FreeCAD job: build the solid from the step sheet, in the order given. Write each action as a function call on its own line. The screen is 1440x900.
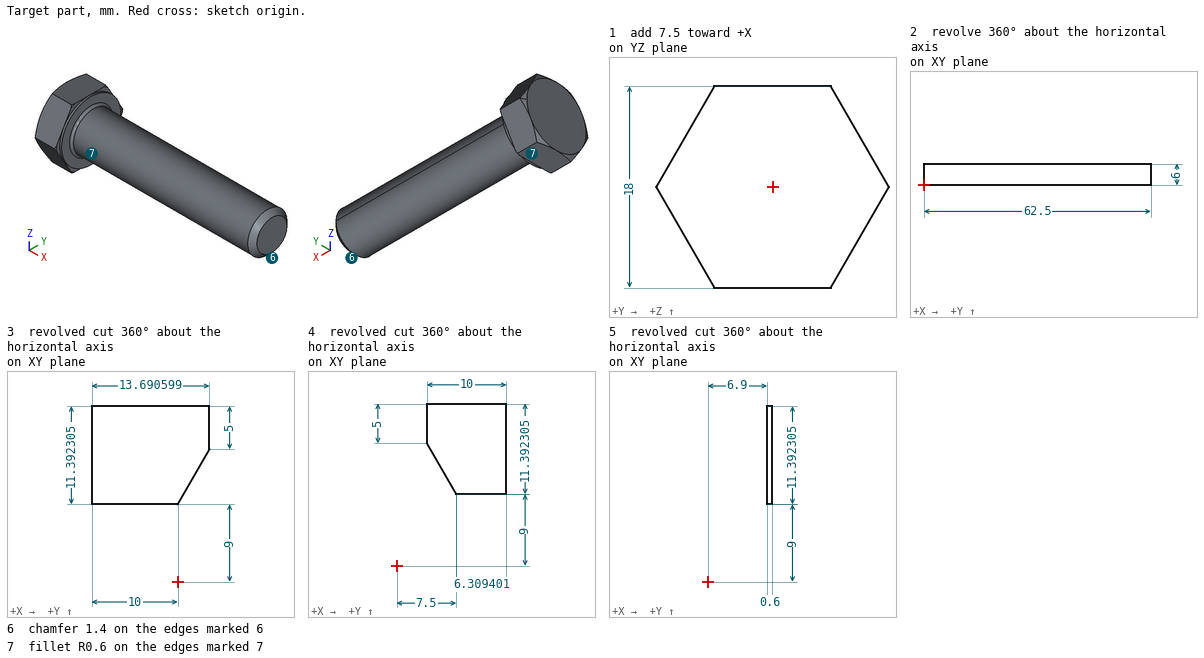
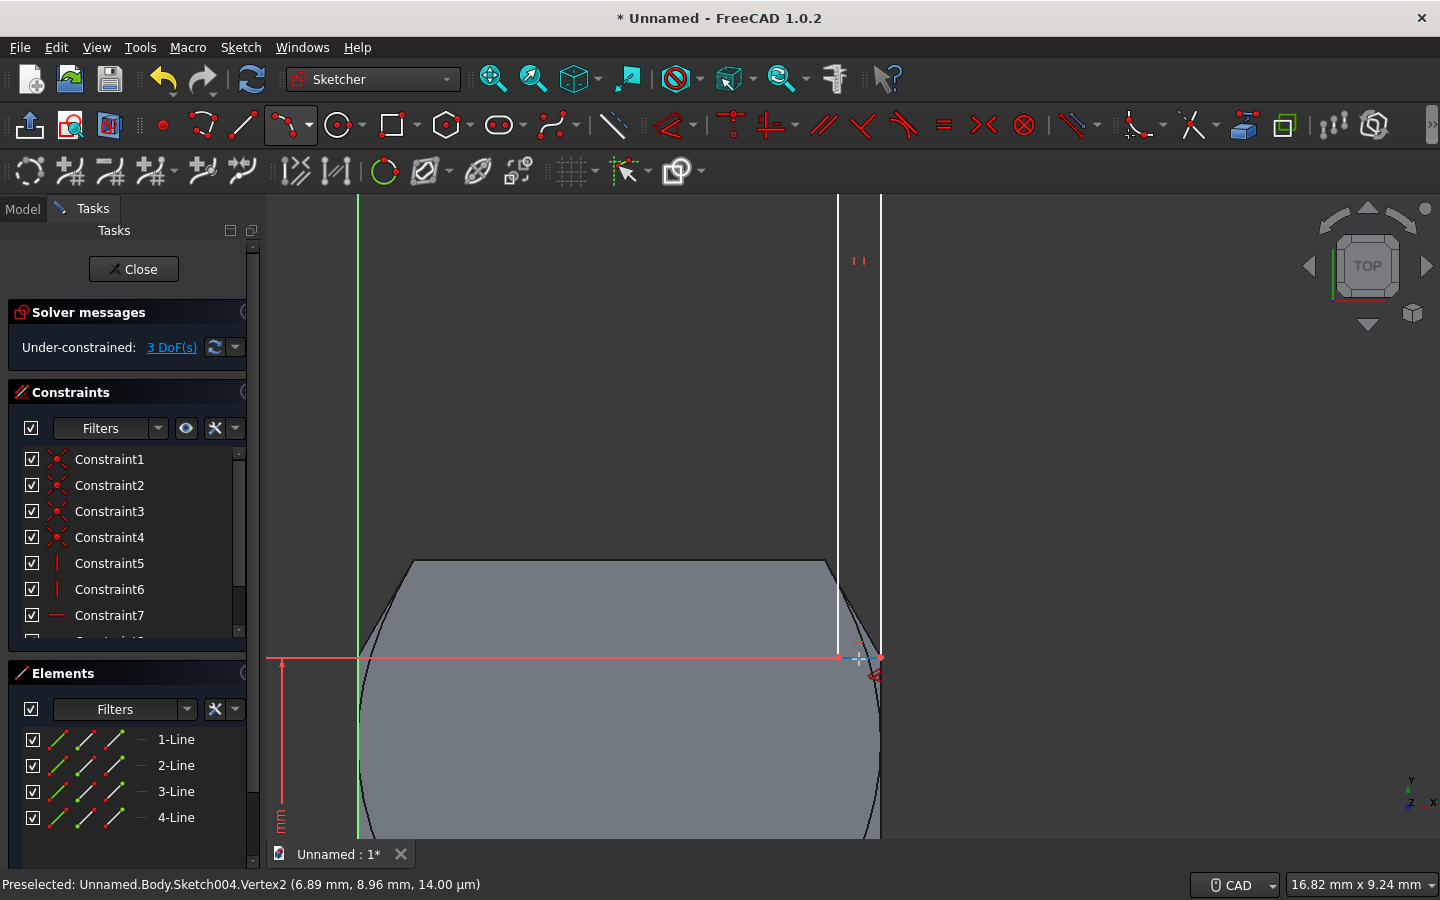
click(859, 658)
click(859, 692)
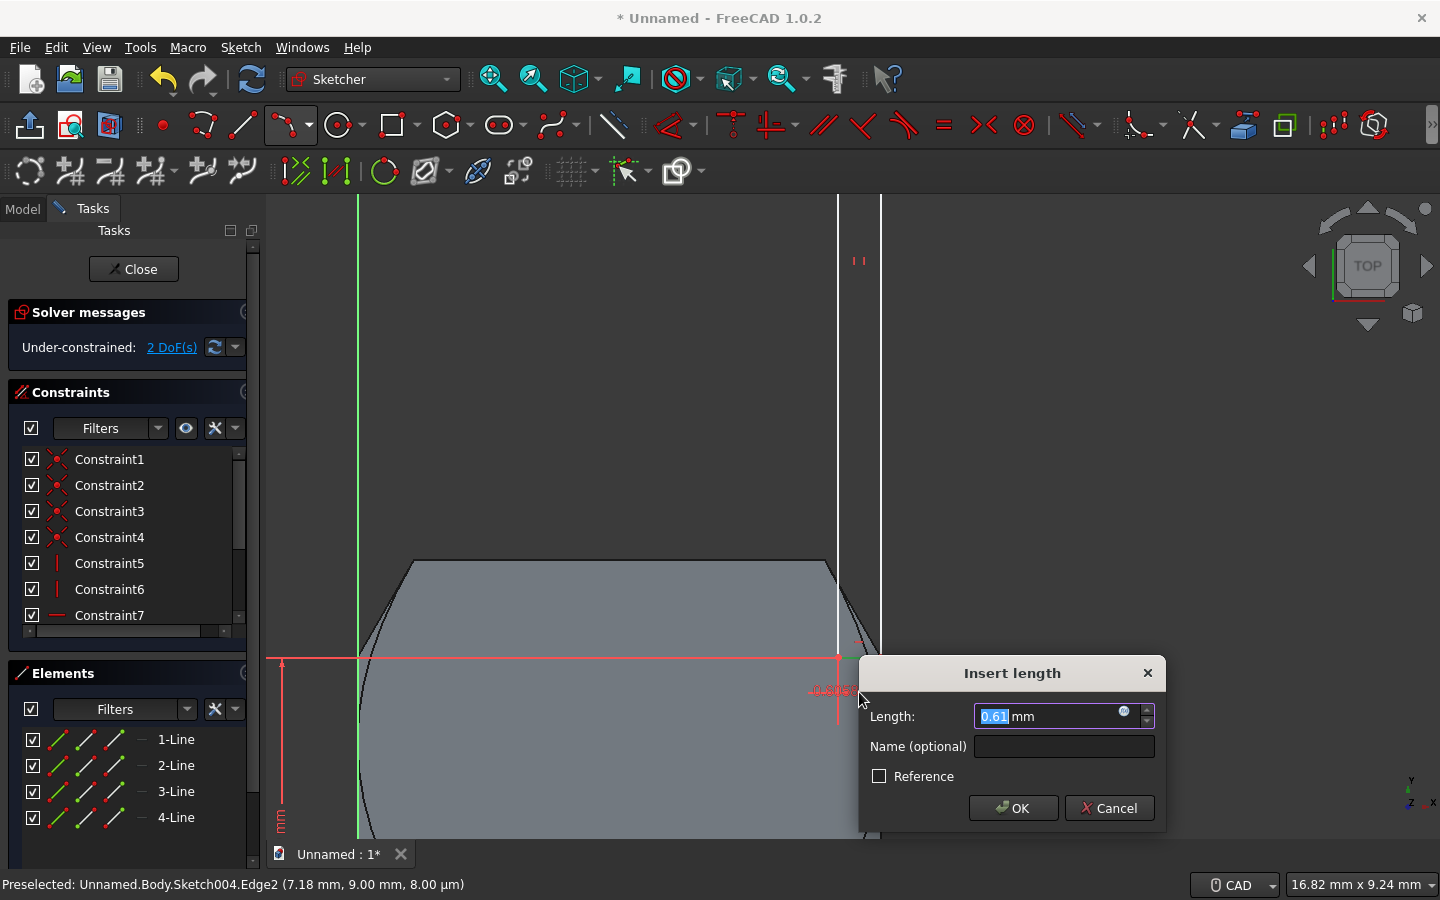
text(0.6)
key(Return)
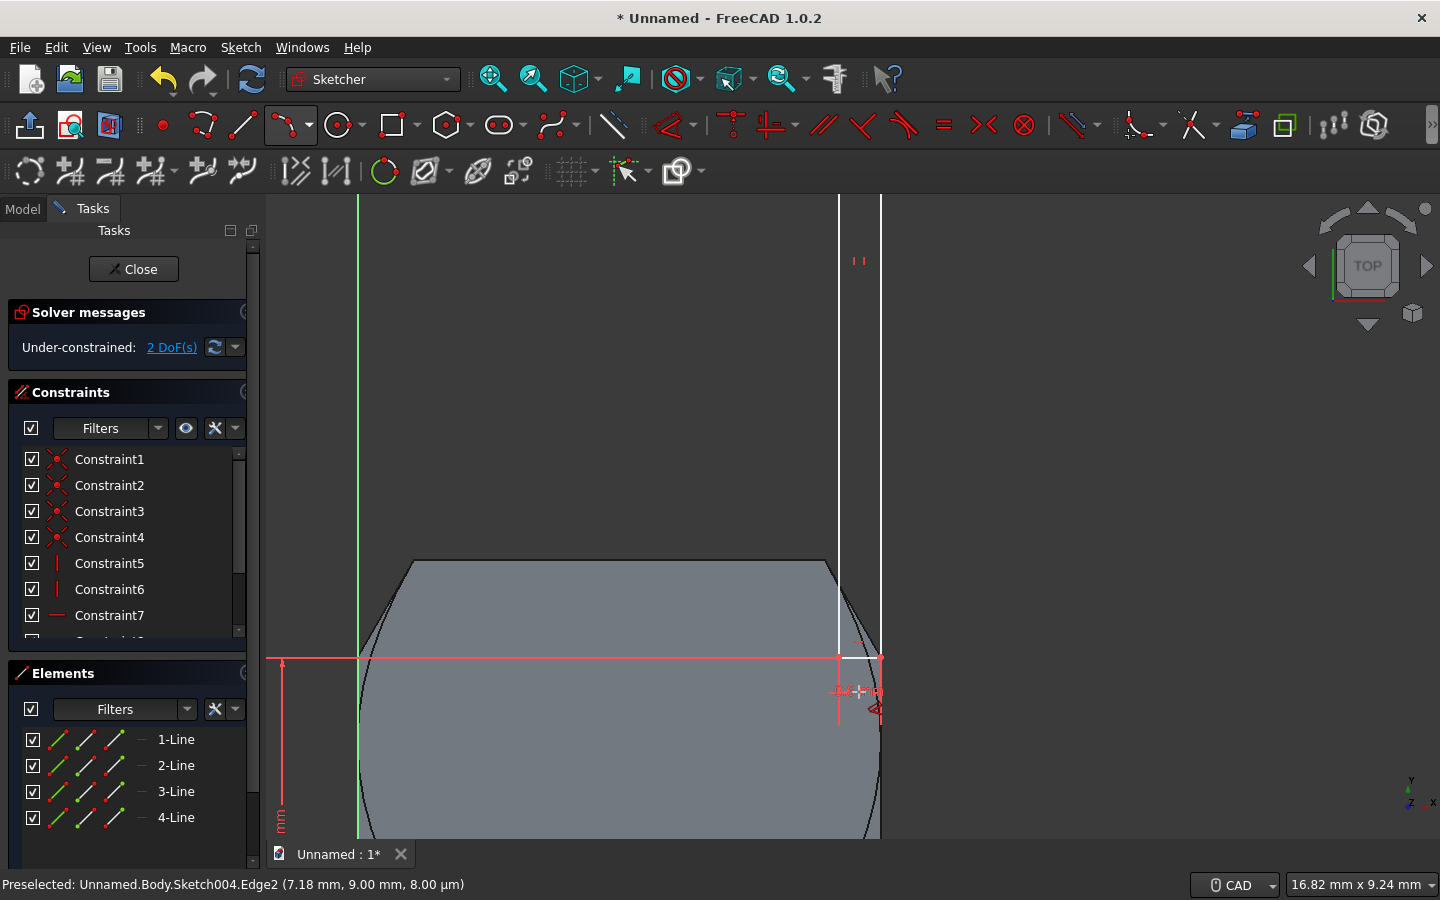
scroll(856, 492, down, 6)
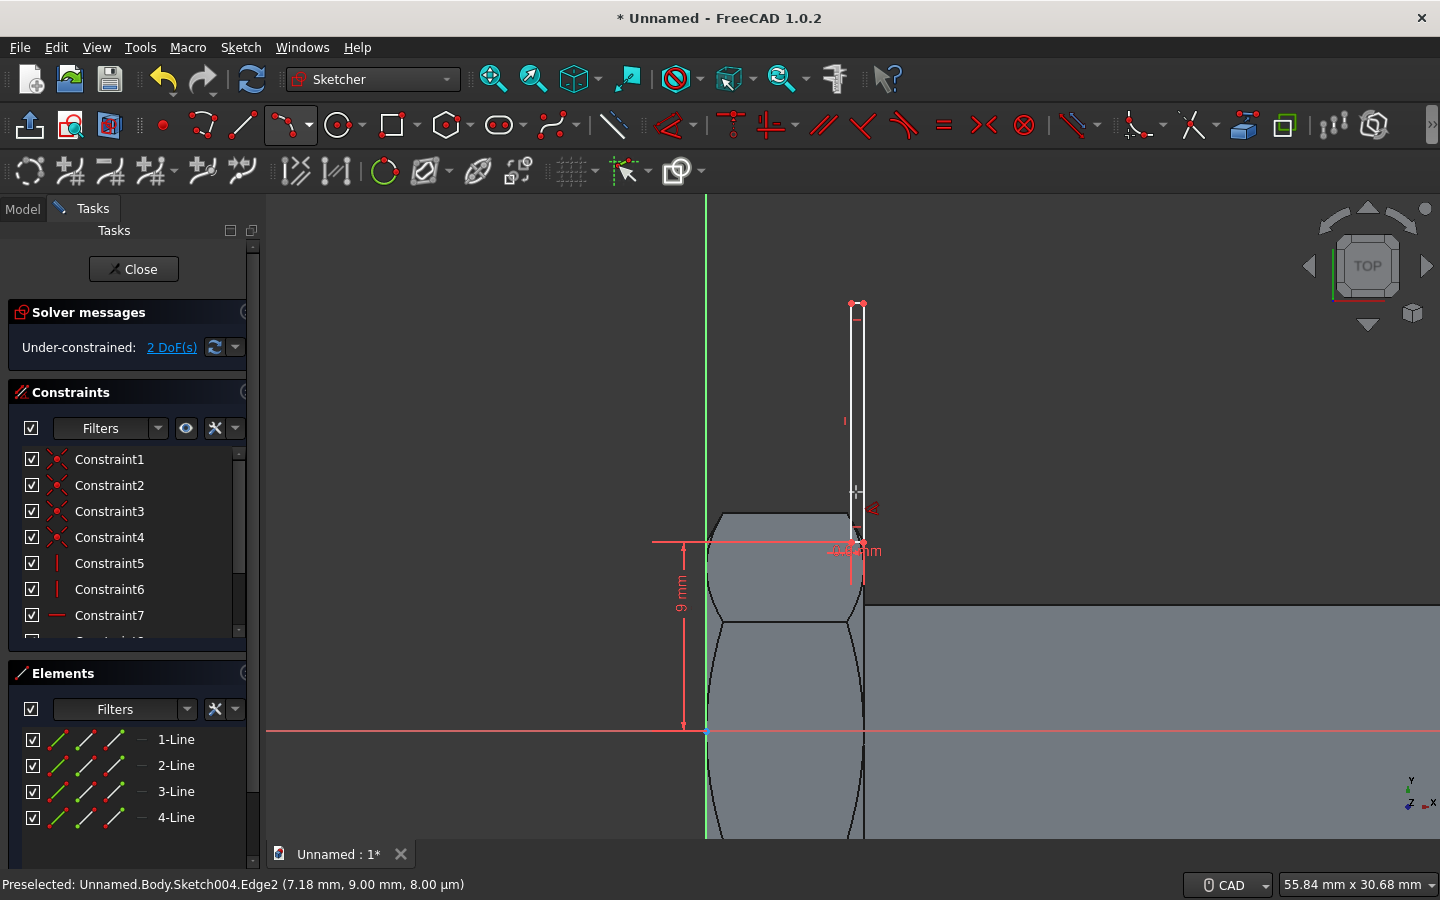
click(851, 303)
click(779, 765)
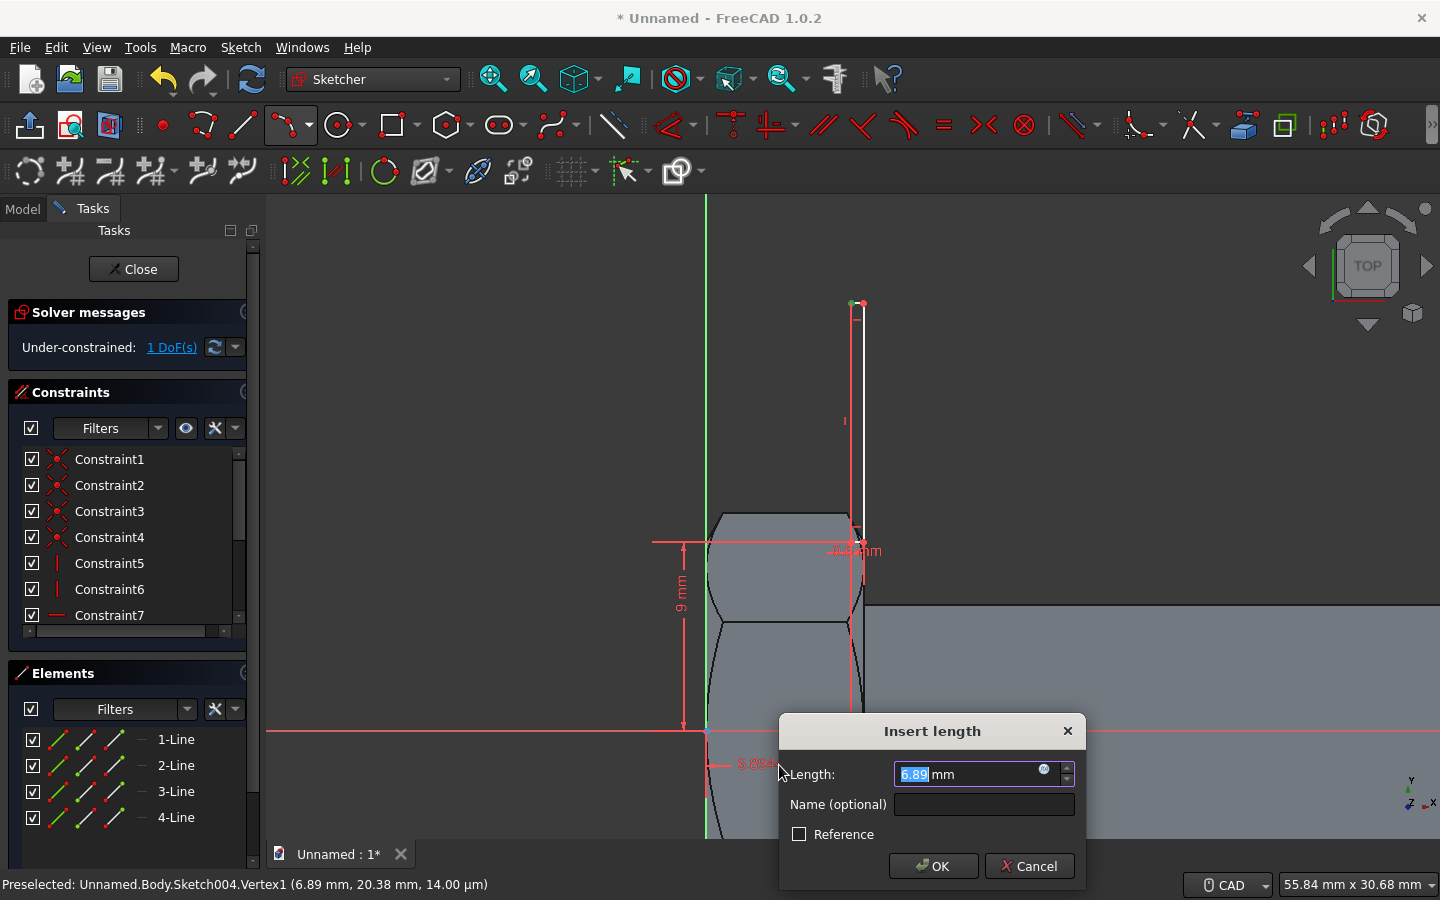
text(6.9)
key(Return)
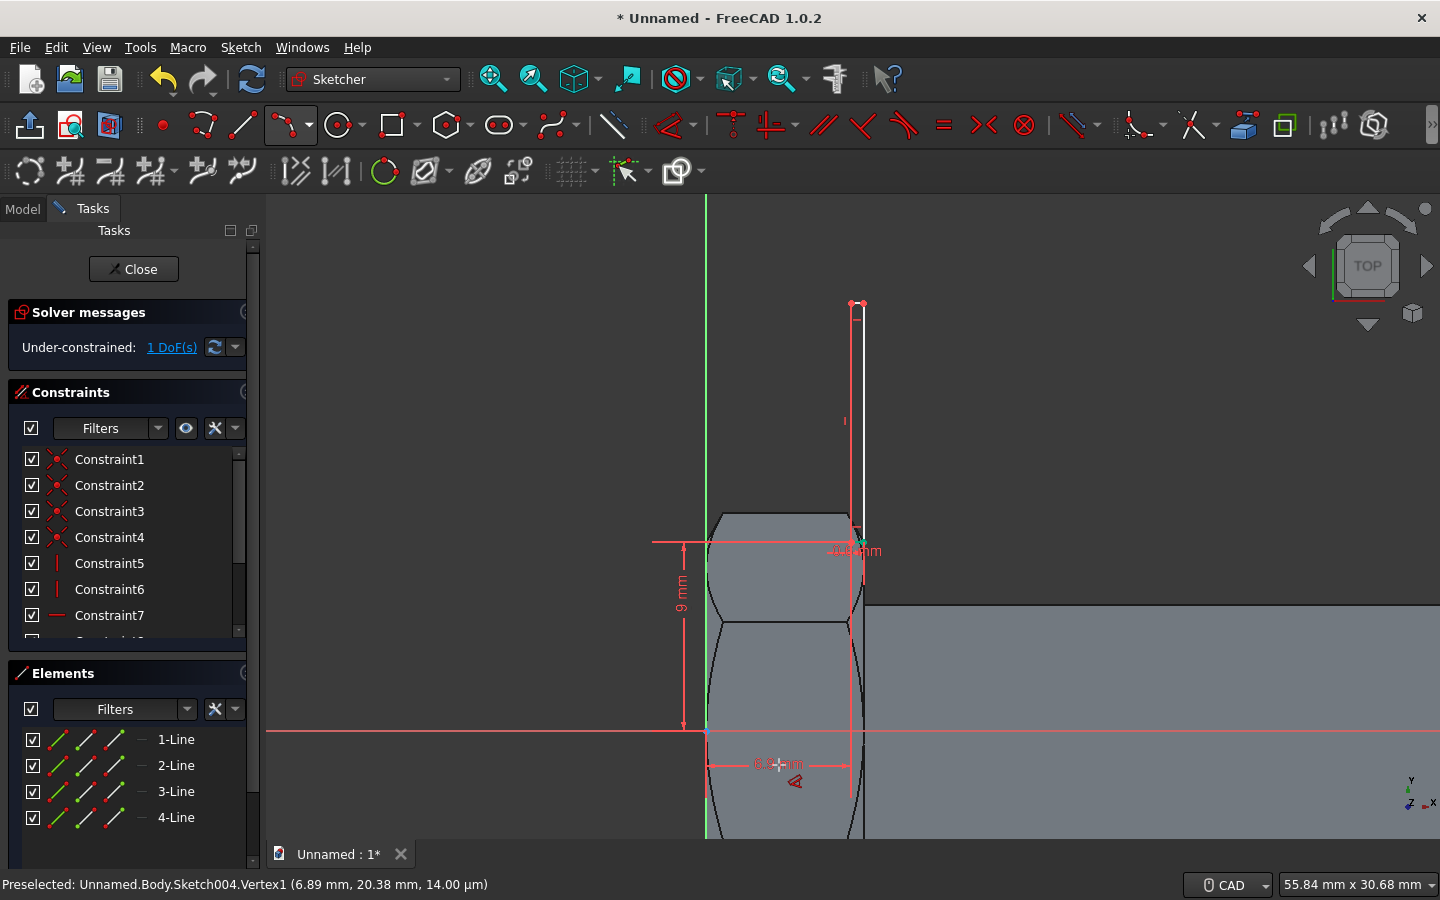
click(851, 375)
click(885, 423)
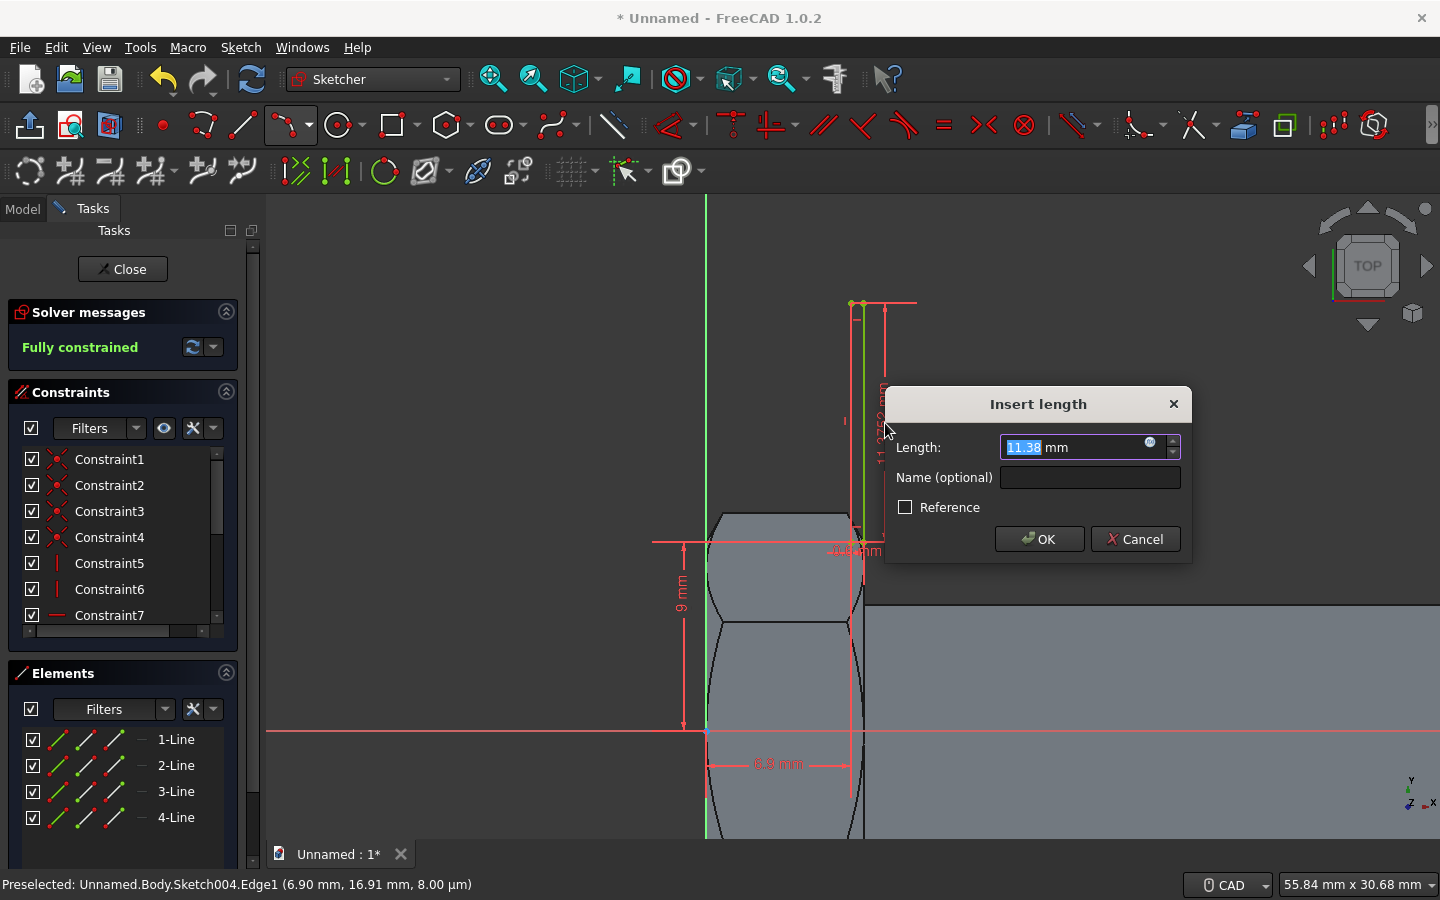
text(11.392305)
key(Return)
key(Escape)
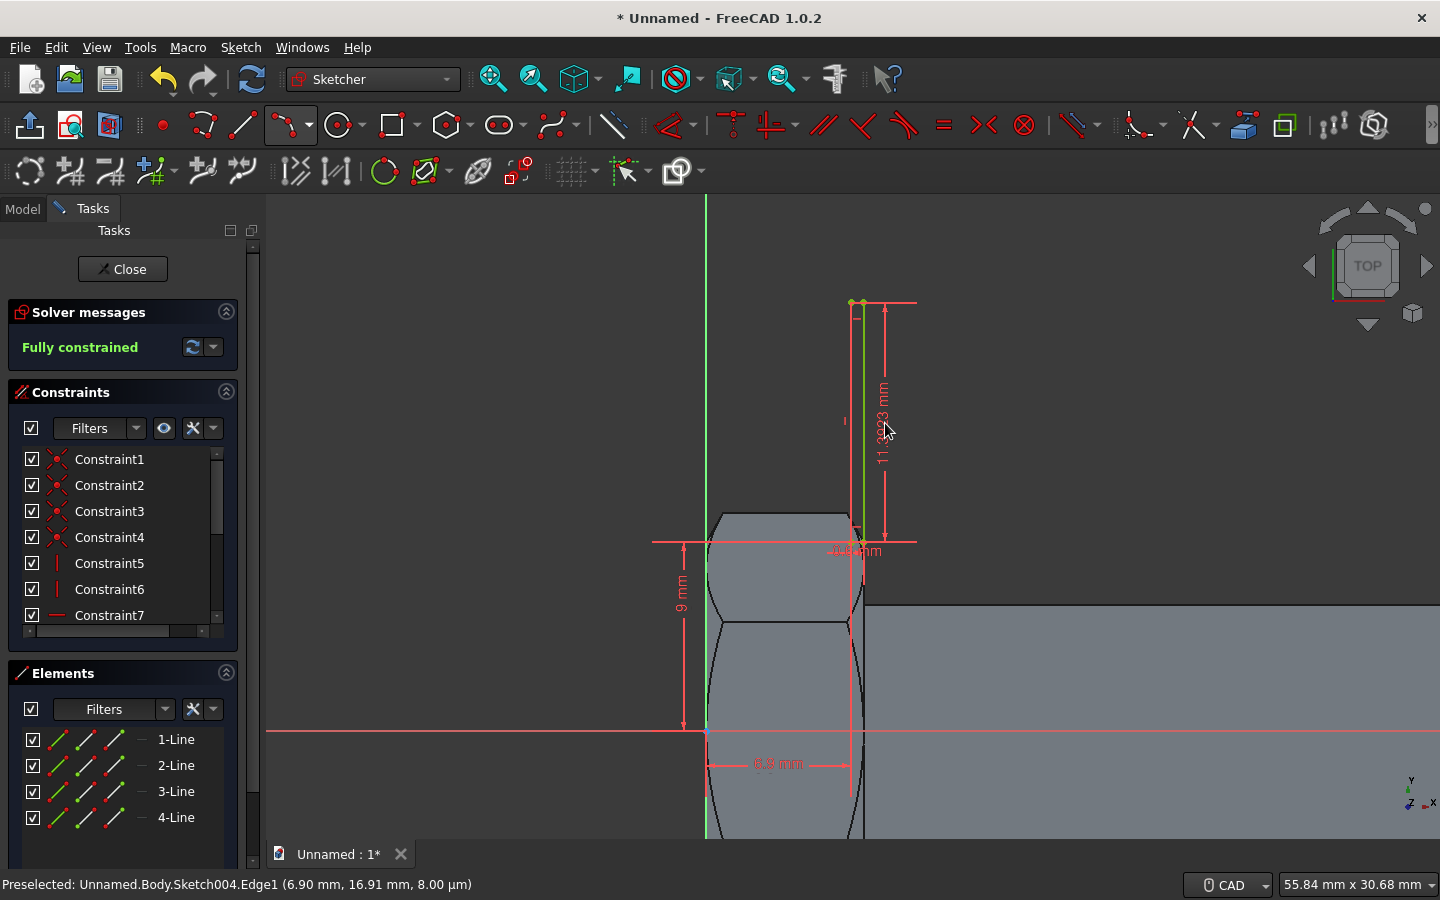
click(123, 269)